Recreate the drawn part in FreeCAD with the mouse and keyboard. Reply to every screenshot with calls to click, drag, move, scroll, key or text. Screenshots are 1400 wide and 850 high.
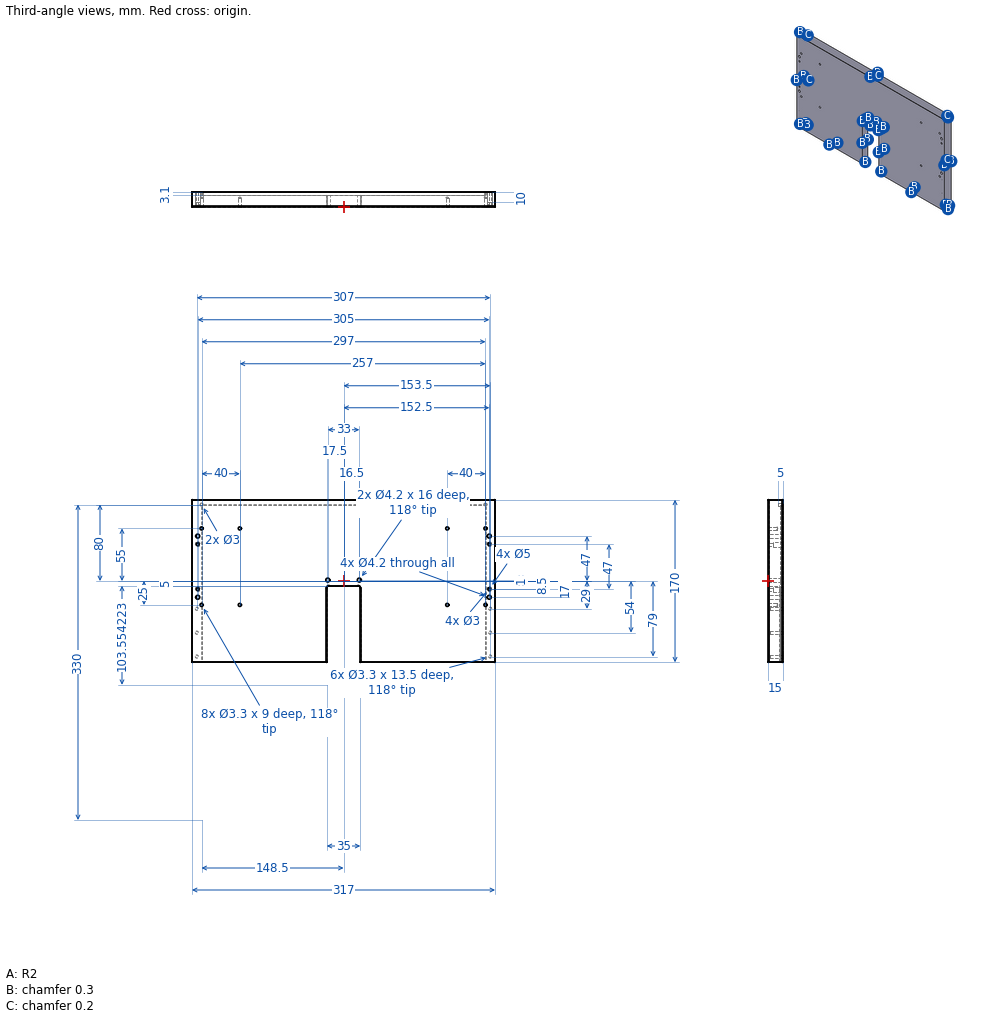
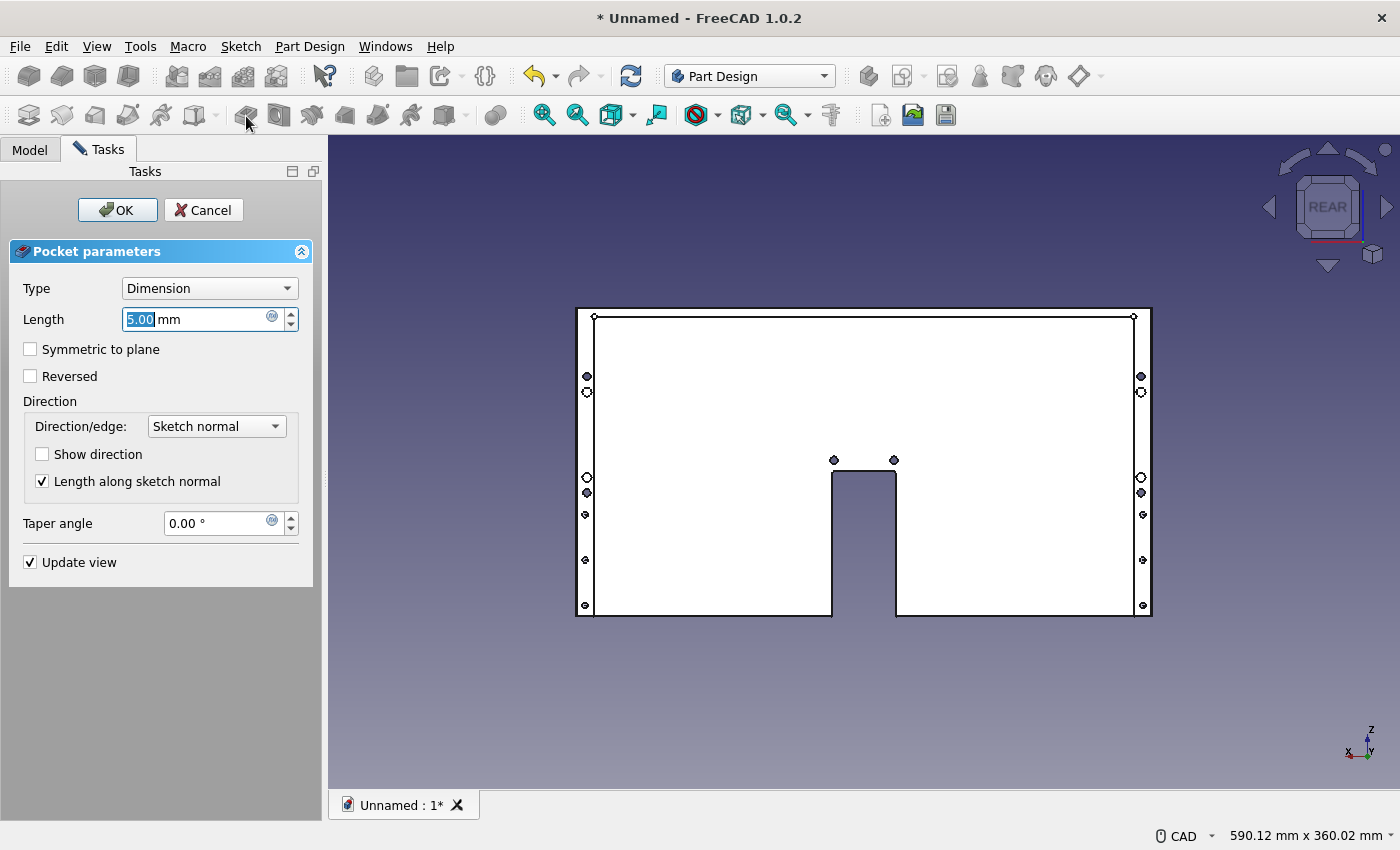
click(210, 288)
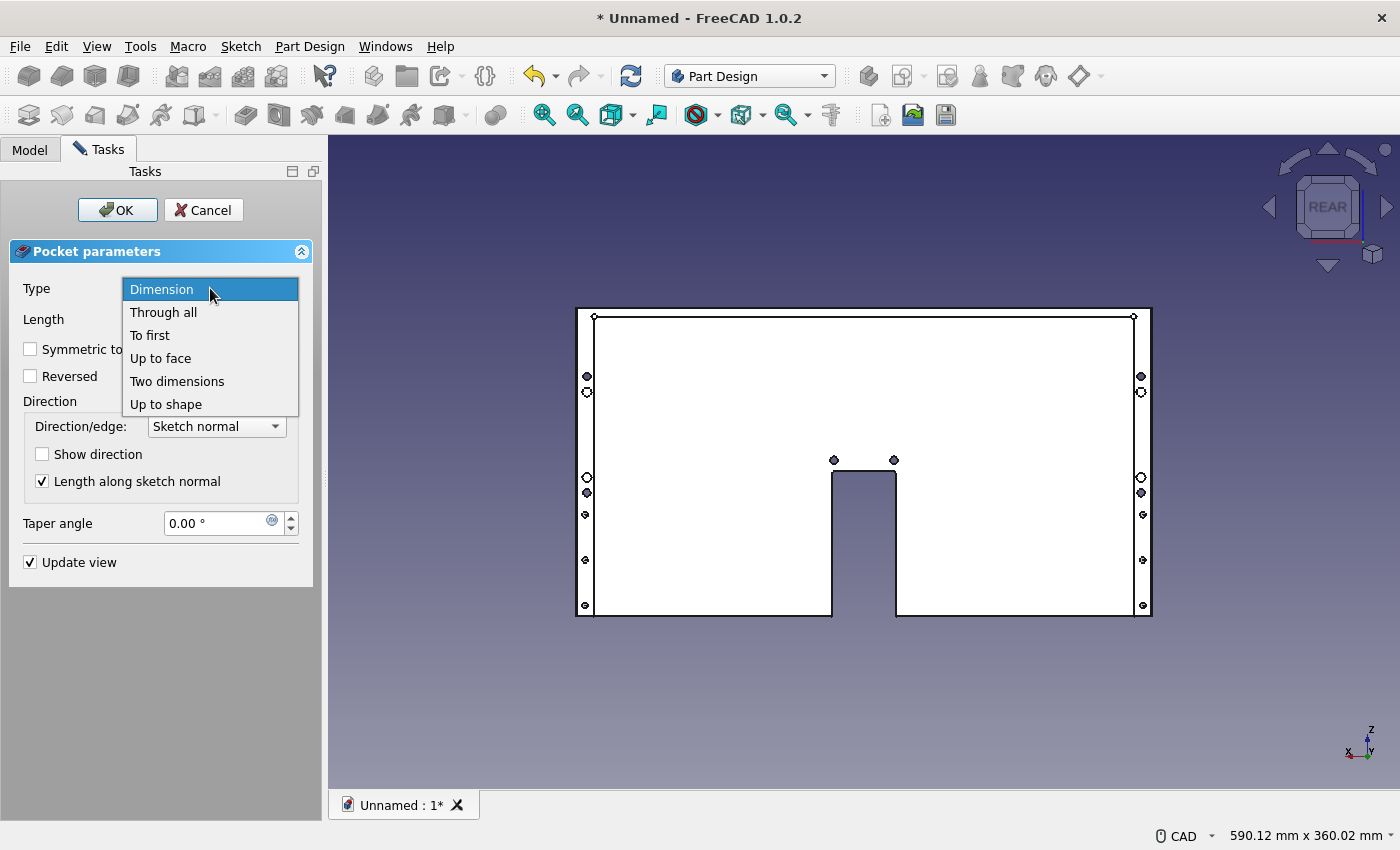
click(208, 312)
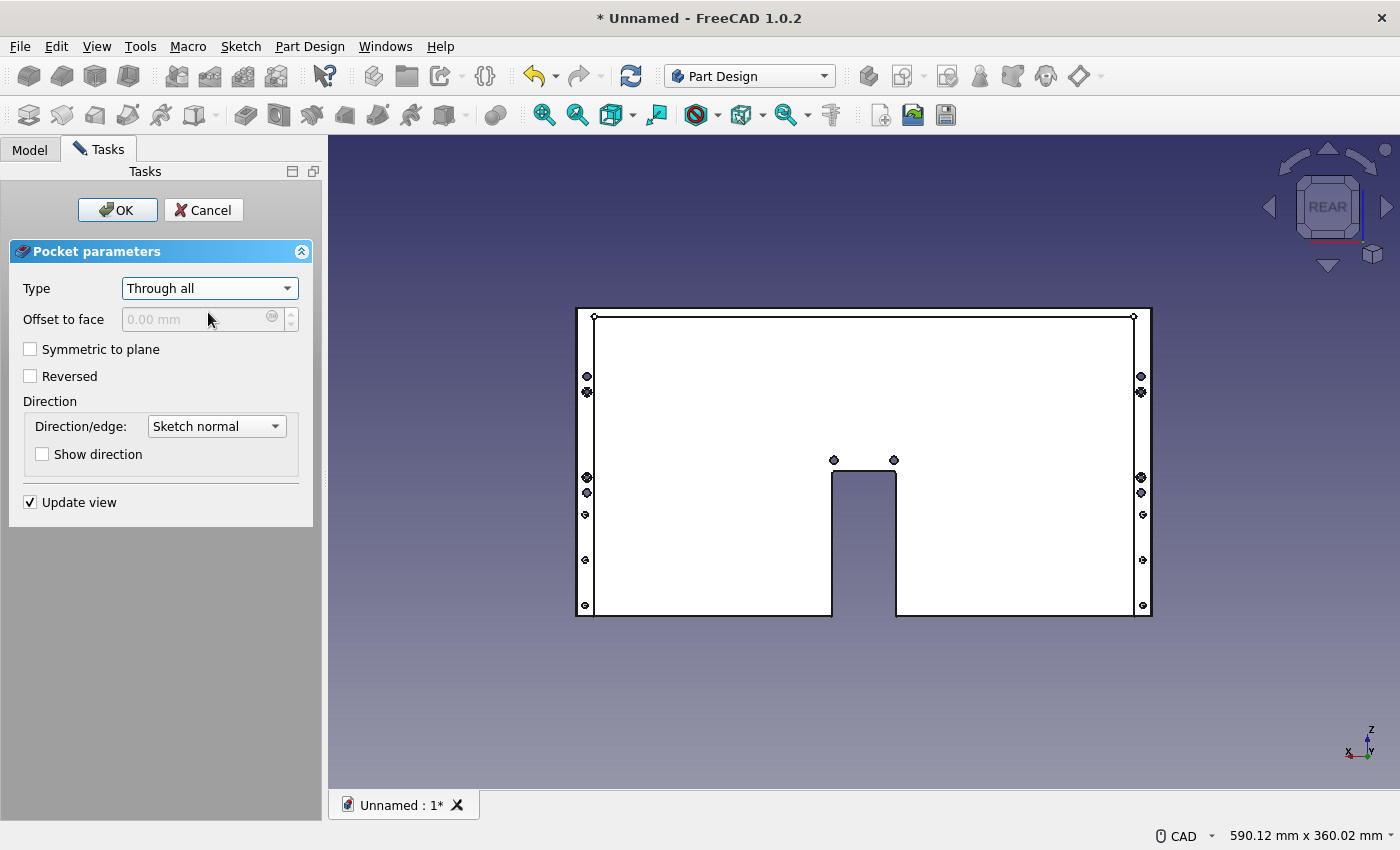
click(118, 210)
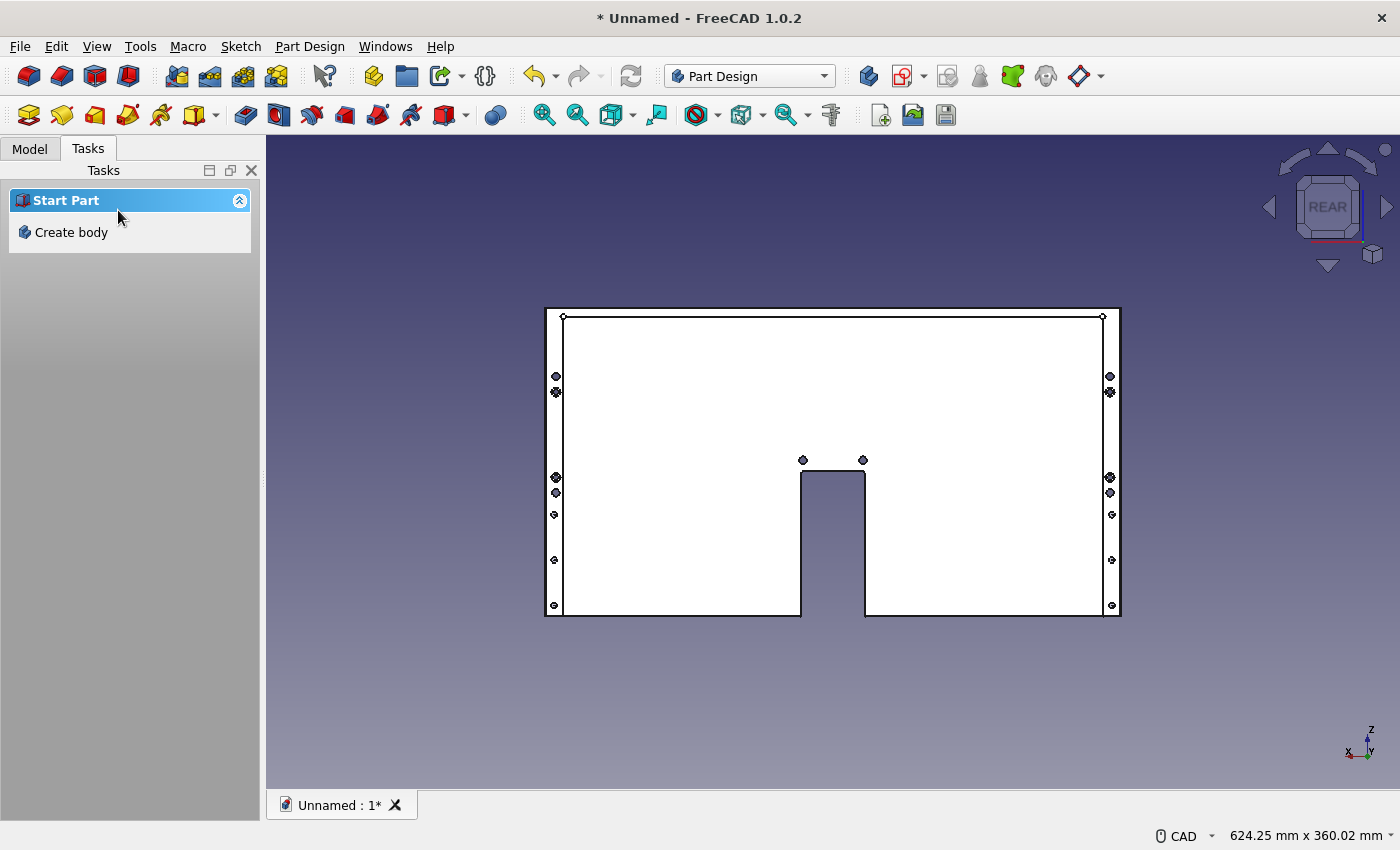
click(902, 76)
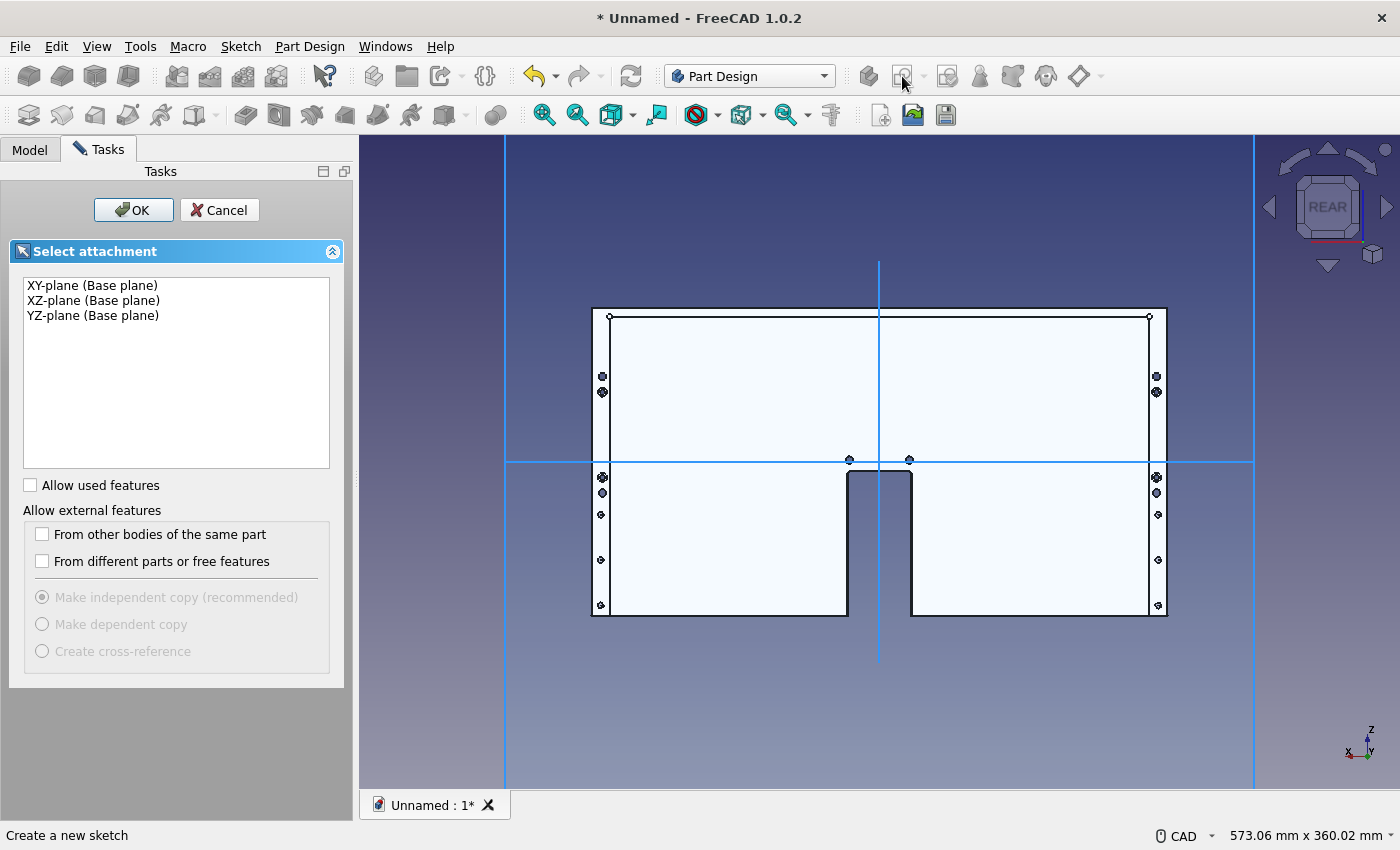
click(84, 300)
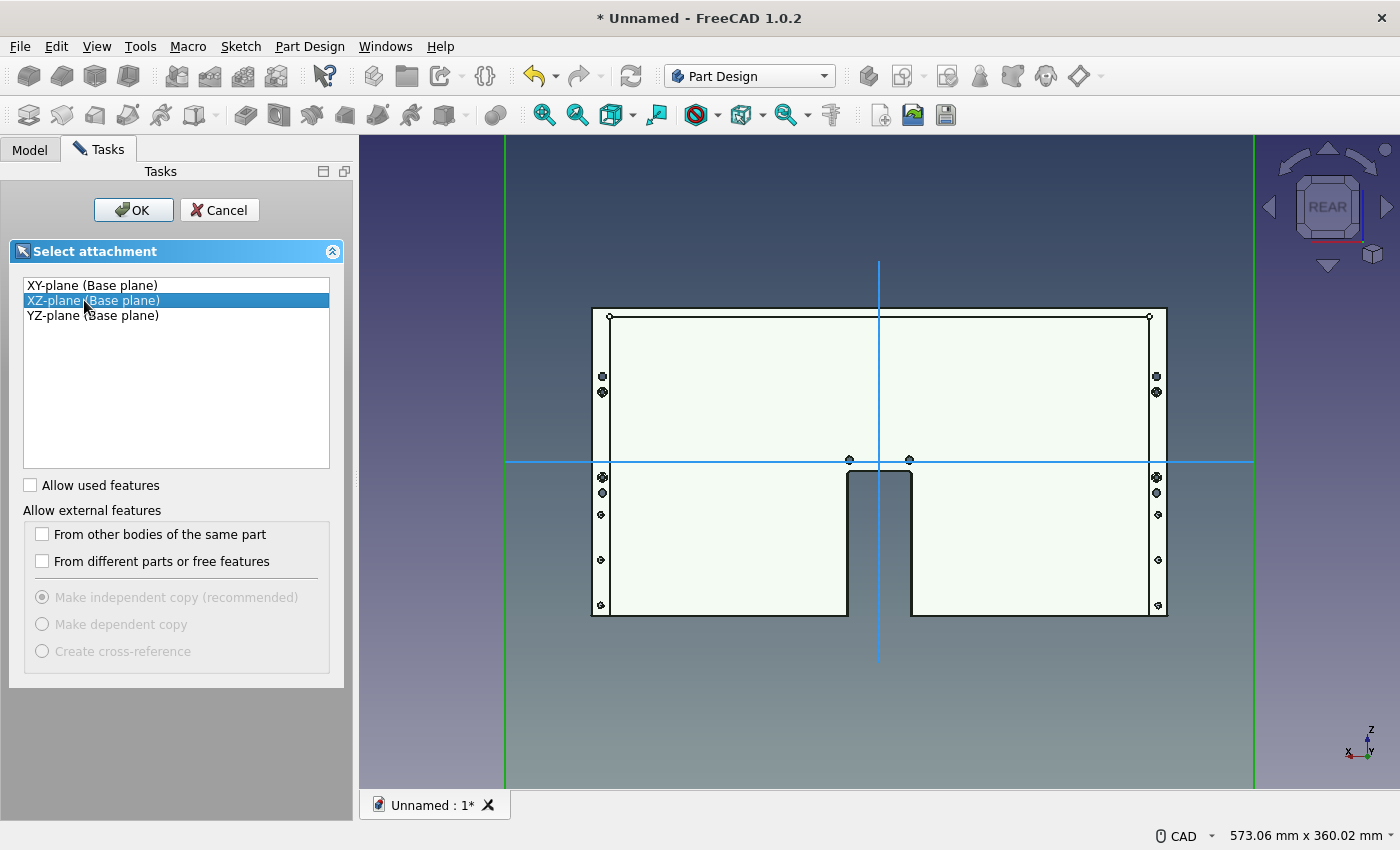
click(134, 210)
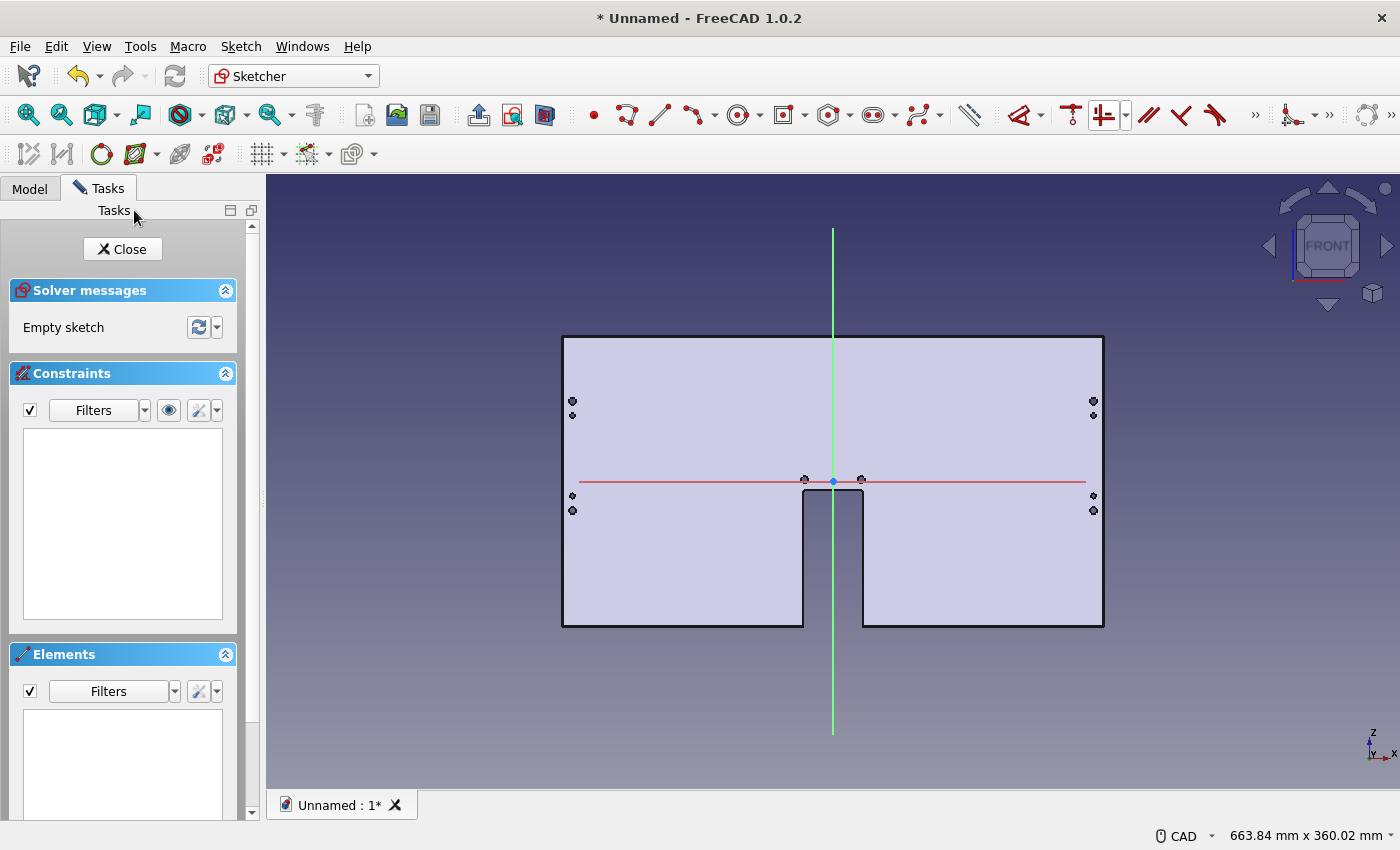
click(738, 116)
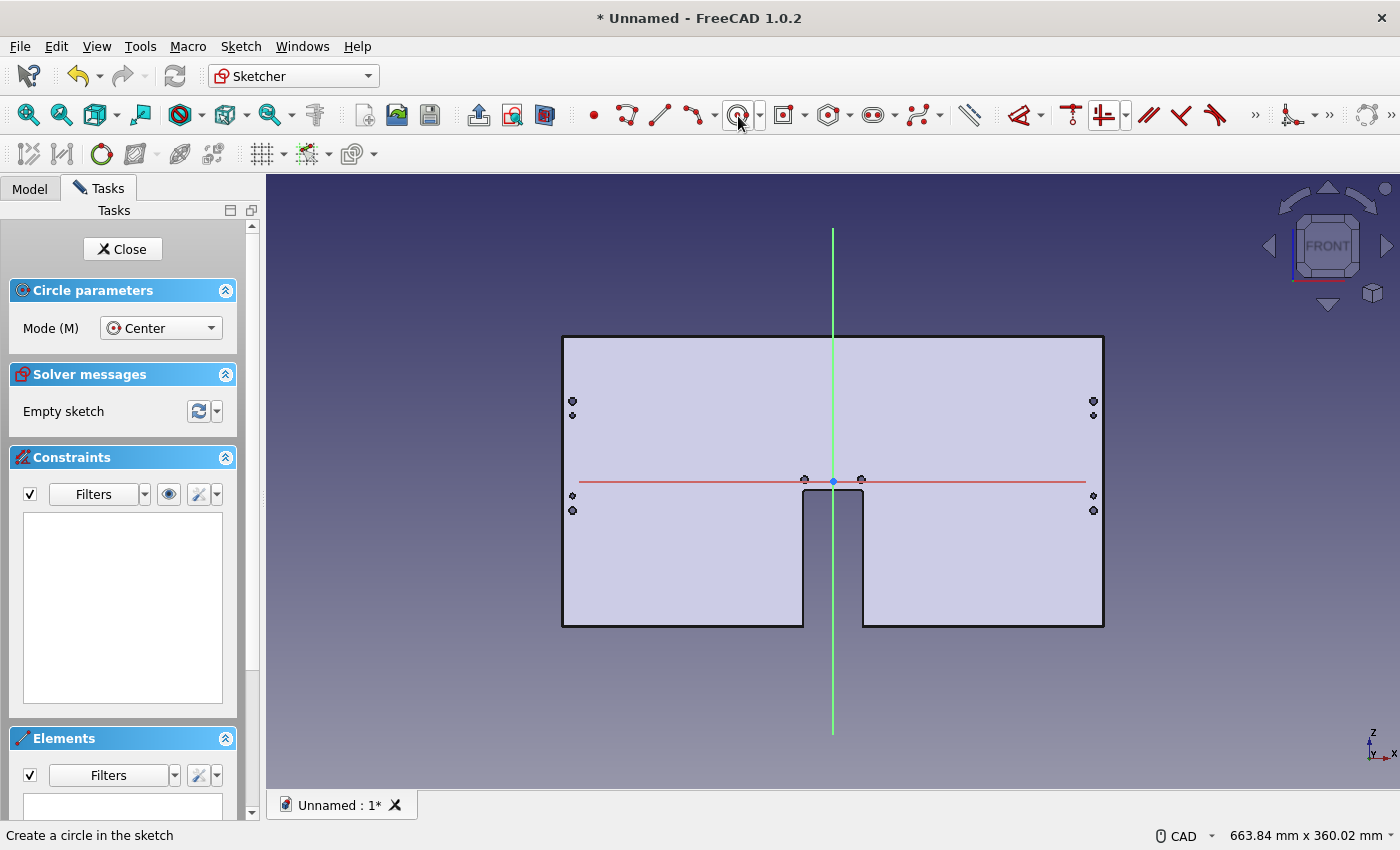
scroll(579, 524, up, 11)